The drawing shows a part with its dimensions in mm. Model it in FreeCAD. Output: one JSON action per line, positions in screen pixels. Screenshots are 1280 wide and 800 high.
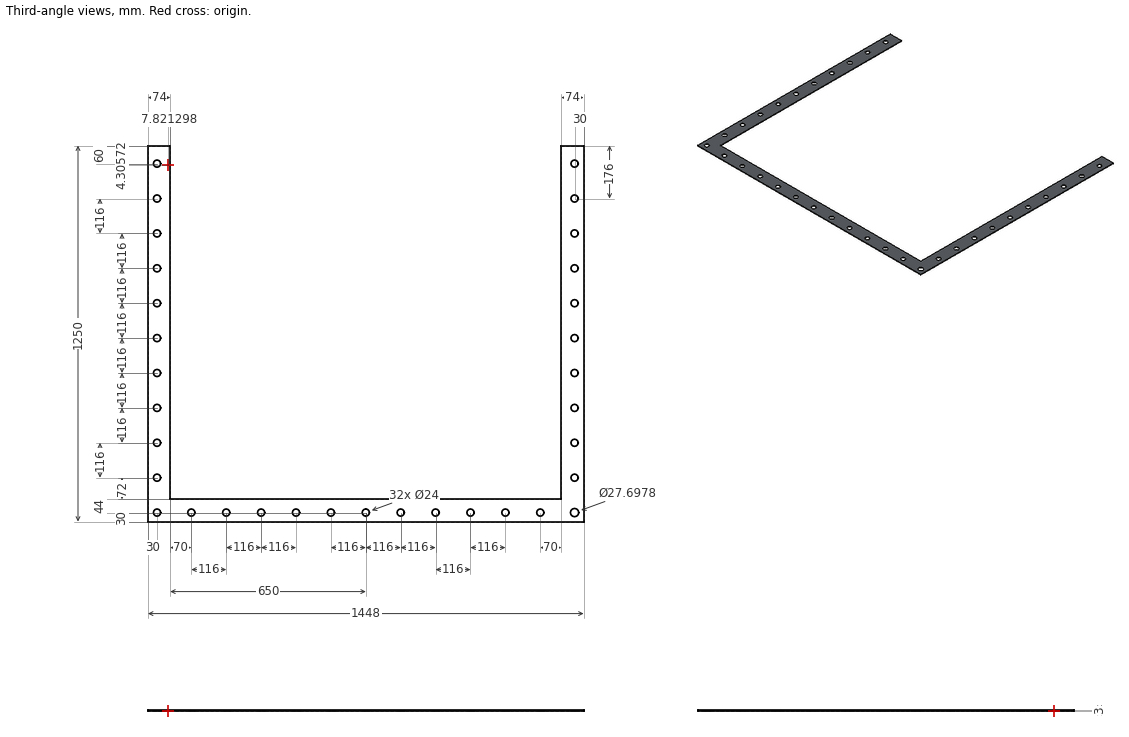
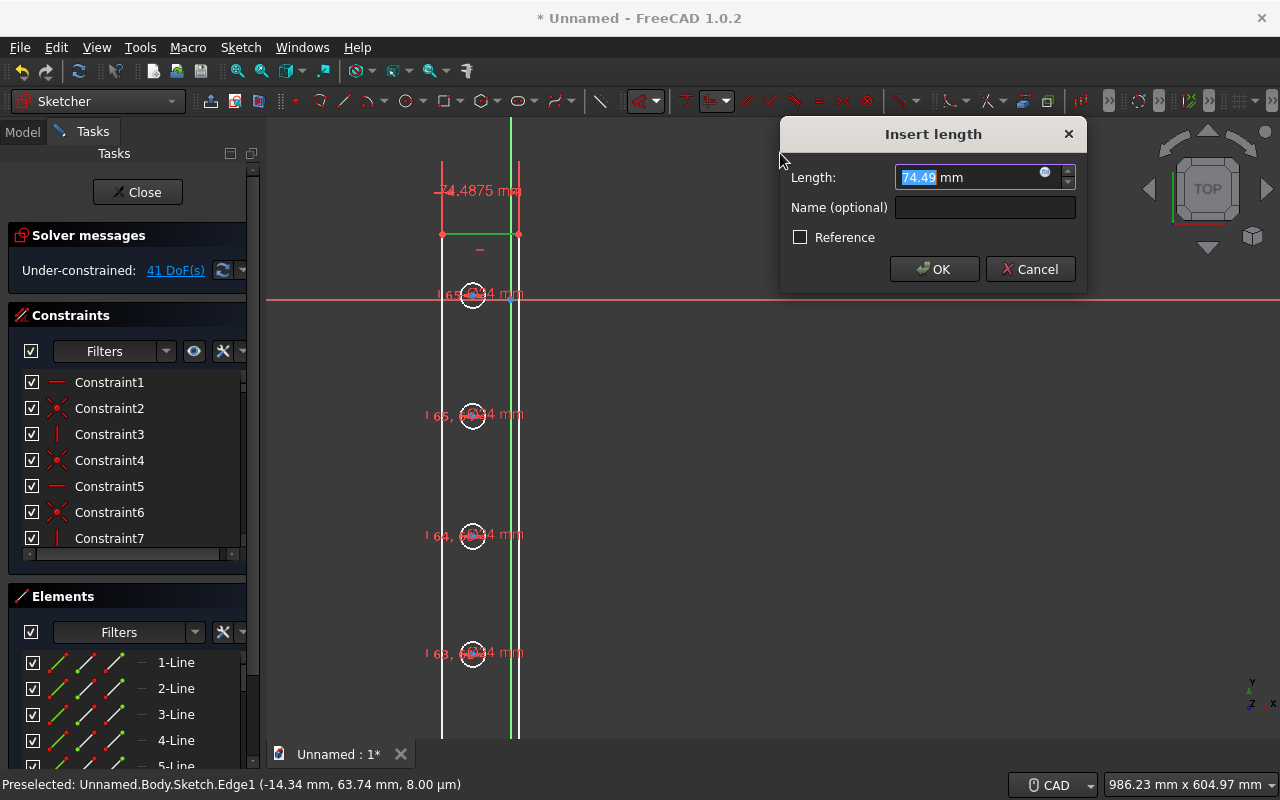
{"action": "type", "text": "74"}
{"action": "key", "text": "Return"}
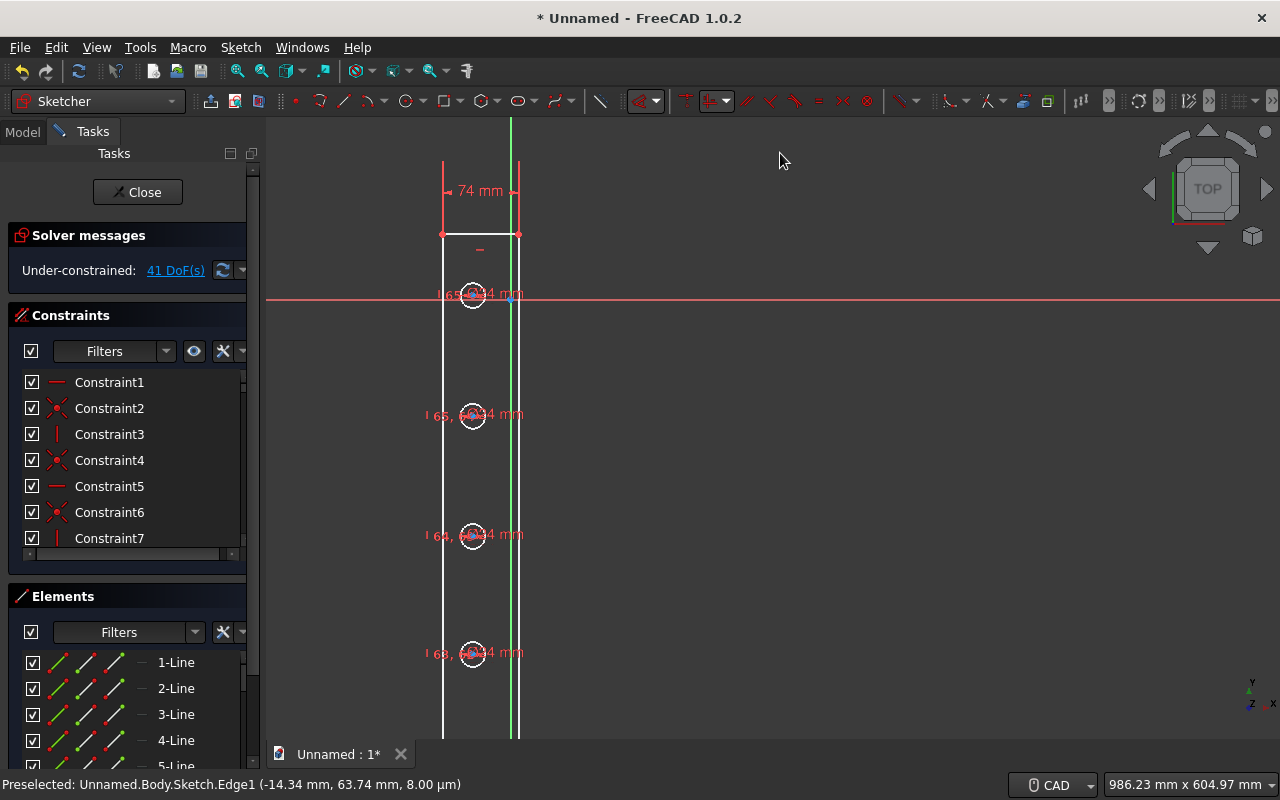
{"action": "scroll", "coordinate": [496, 235], "scroll_direction": "down", "scroll_amount": 6}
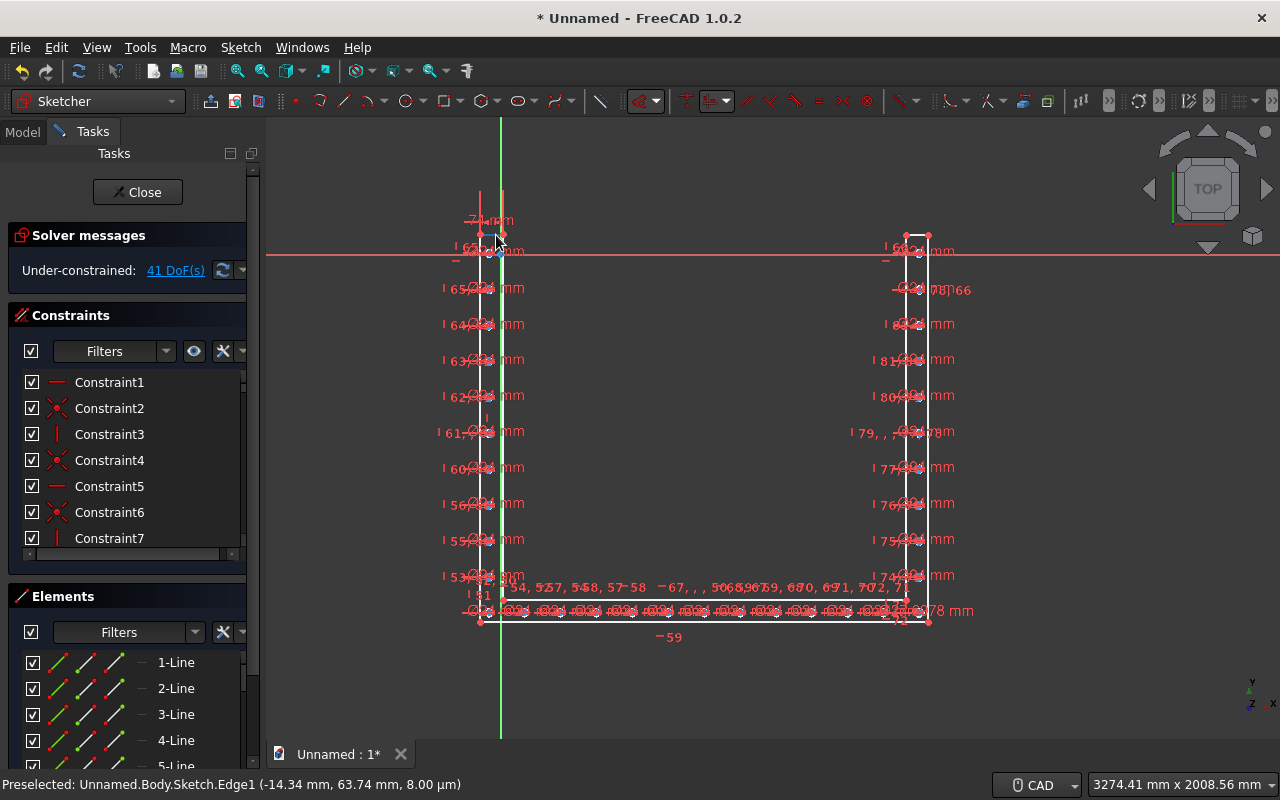
{"action": "scroll", "coordinate": [921, 235], "scroll_direction": "up", "scroll_amount": 4}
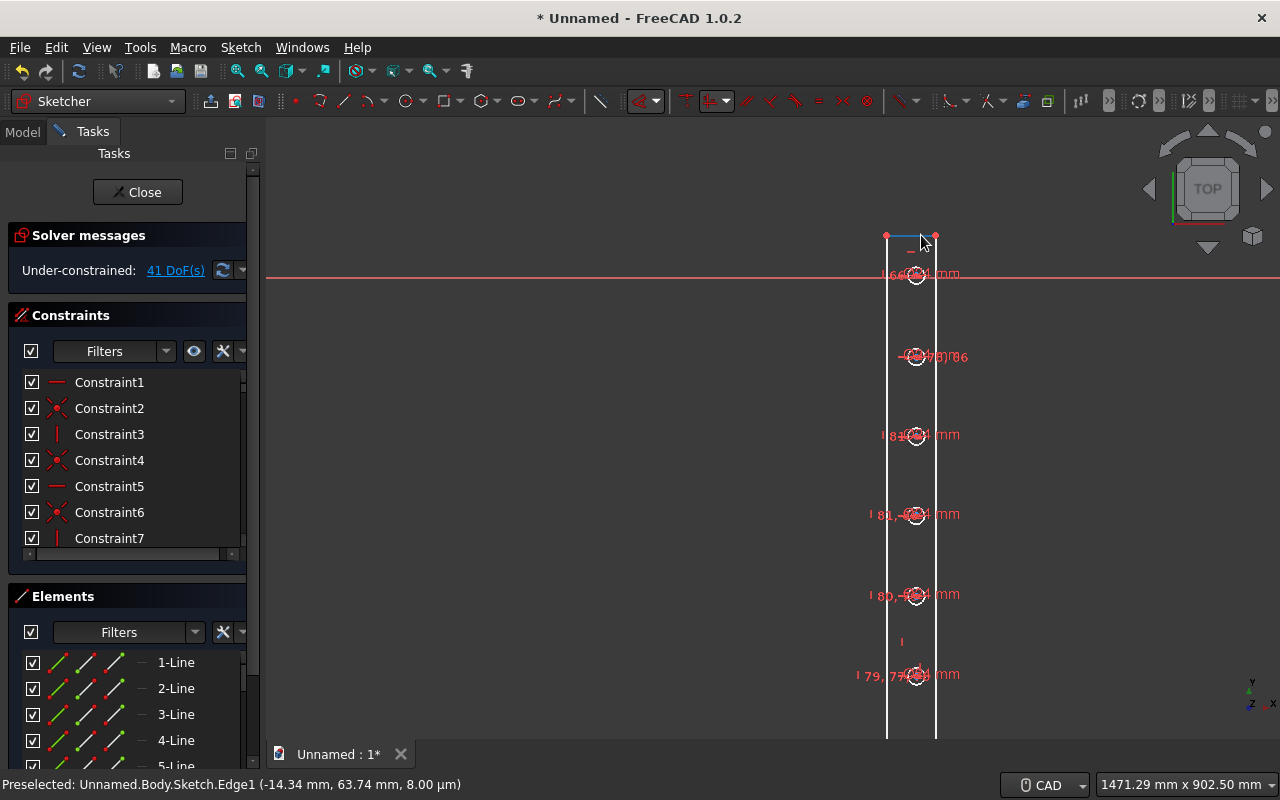
{"action": "left_click", "coordinate": [921, 236]}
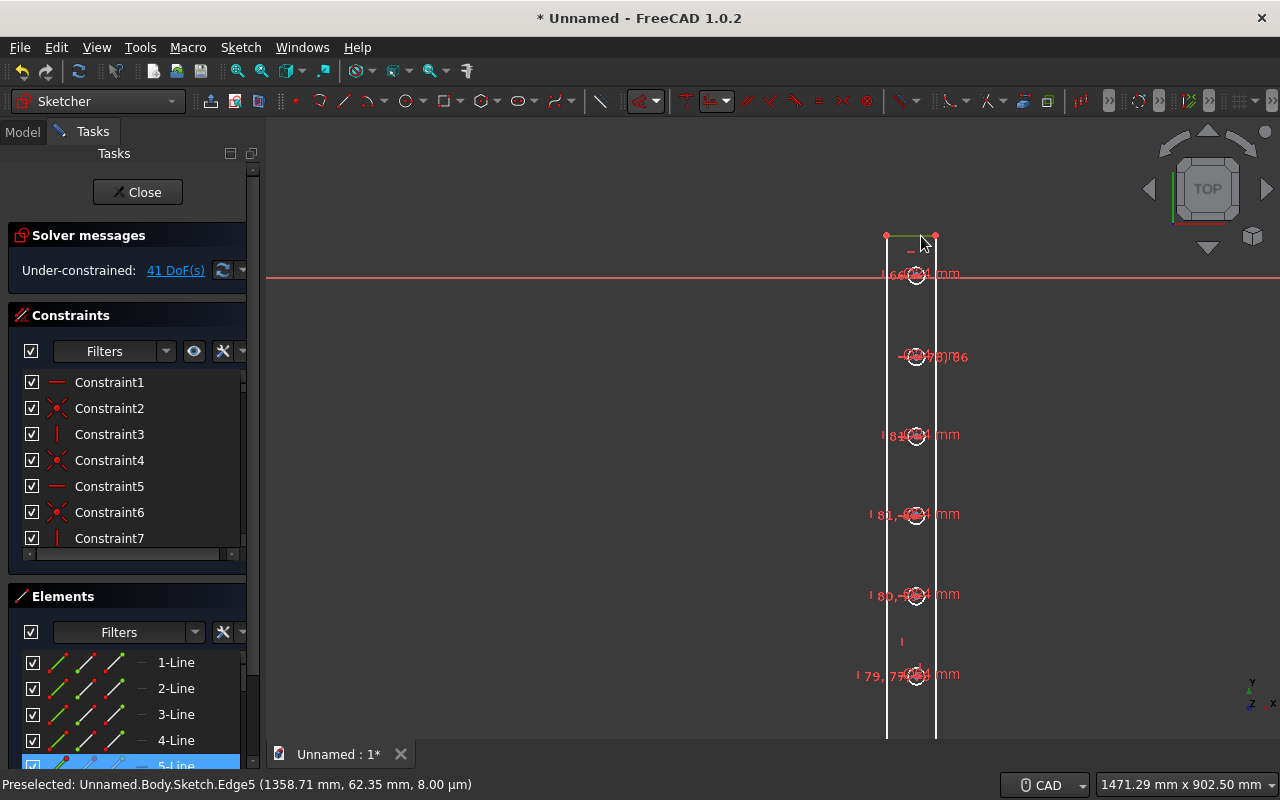
{"action": "key", "text": "l"}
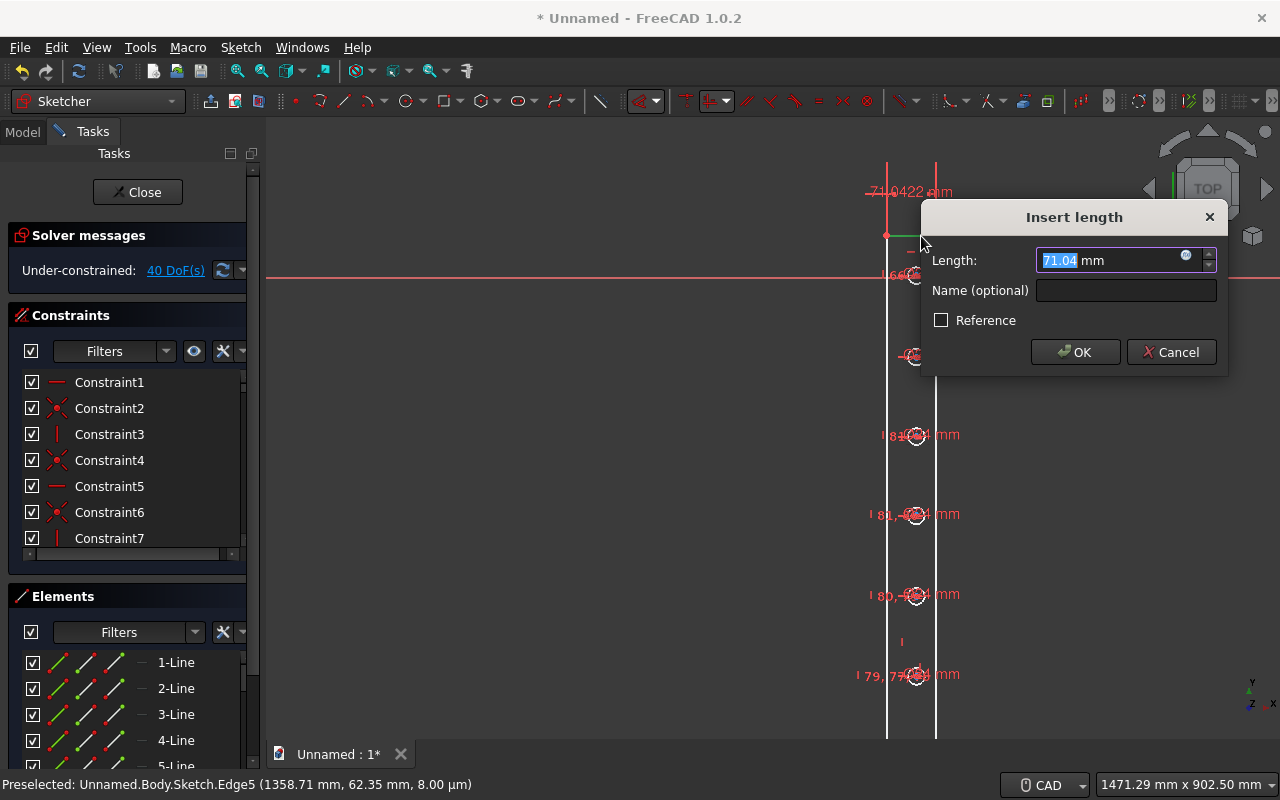
{"action": "type", "text": "74"}
{"action": "key", "text": "Return"}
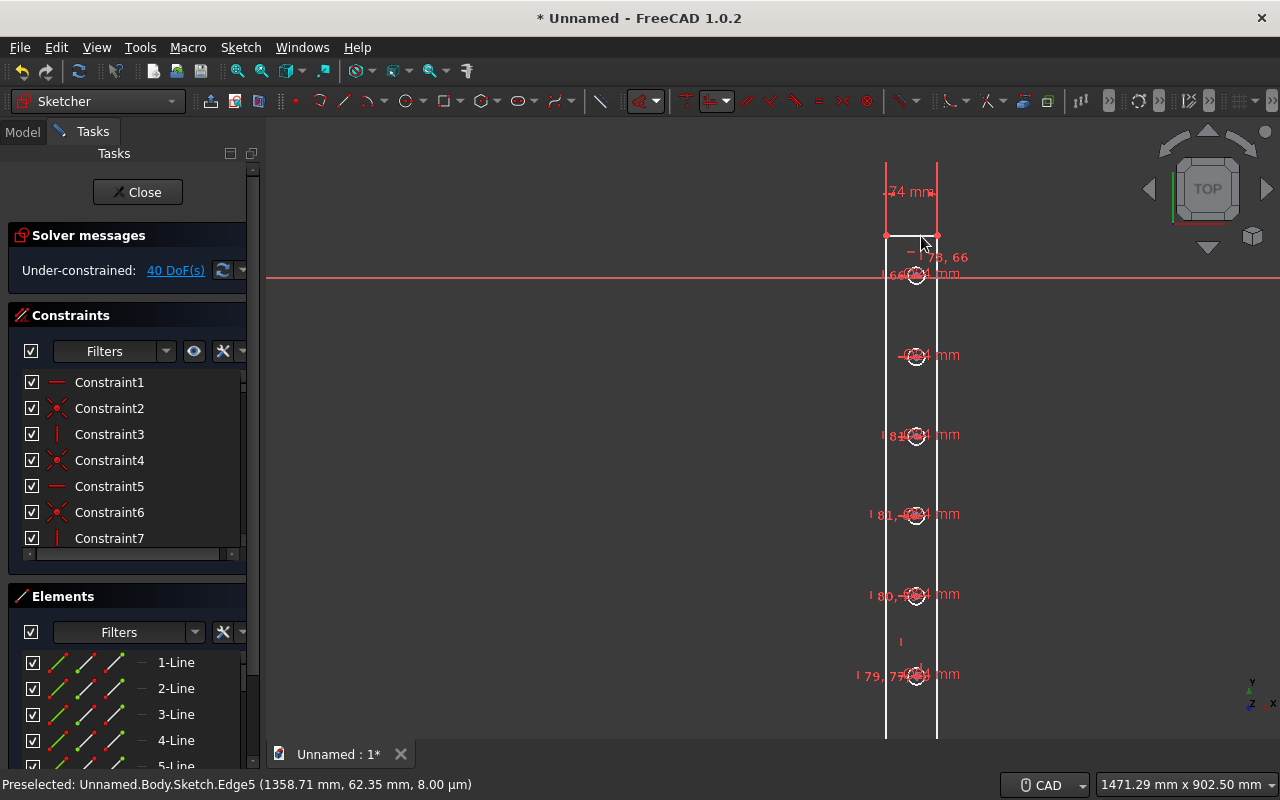
{"action": "scroll", "coordinate": [922, 235], "scroll_direction": "down", "scroll_amount": 4}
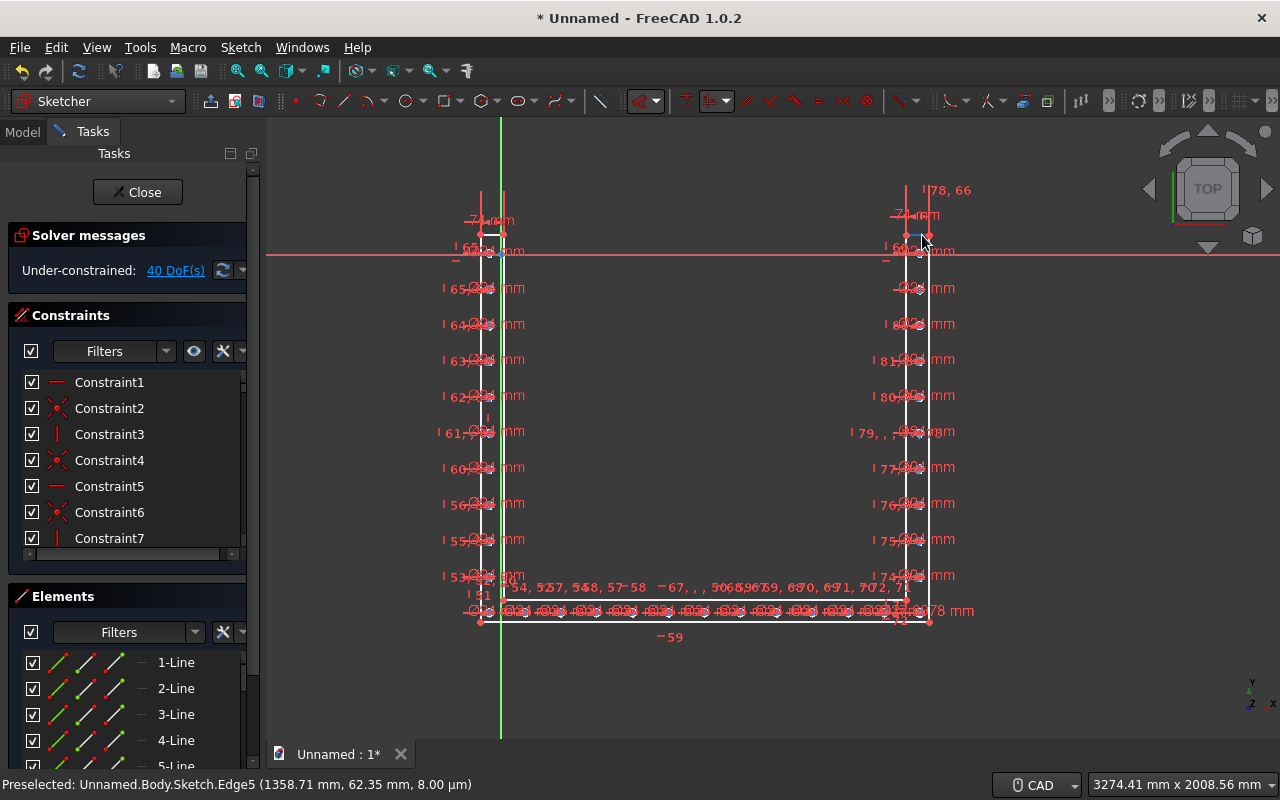
{"action": "scroll", "coordinate": [504, 600], "scroll_direction": "up", "scroll_amount": 6}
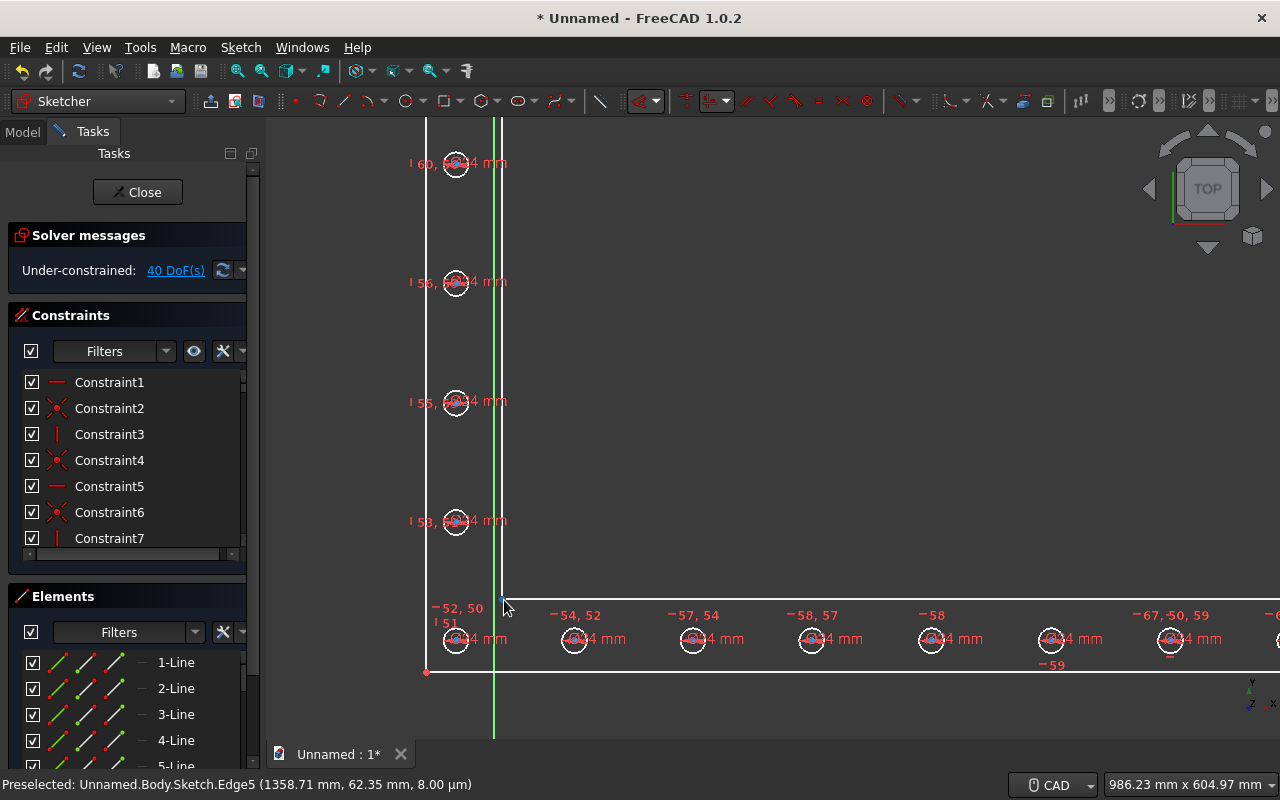
{"action": "left_click", "coordinate": [502, 599]}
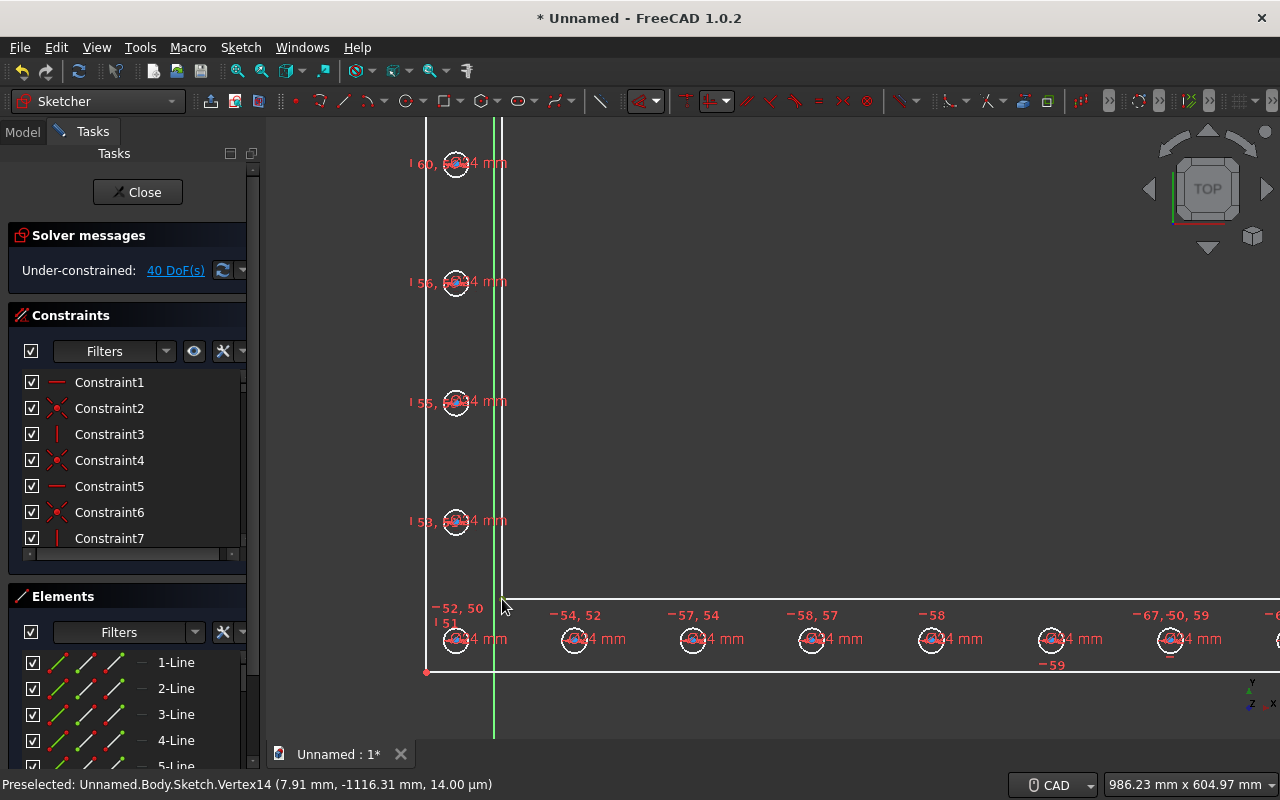
{"action": "scroll", "coordinate": [504, 600], "scroll_direction": "down", "scroll_amount": 6}